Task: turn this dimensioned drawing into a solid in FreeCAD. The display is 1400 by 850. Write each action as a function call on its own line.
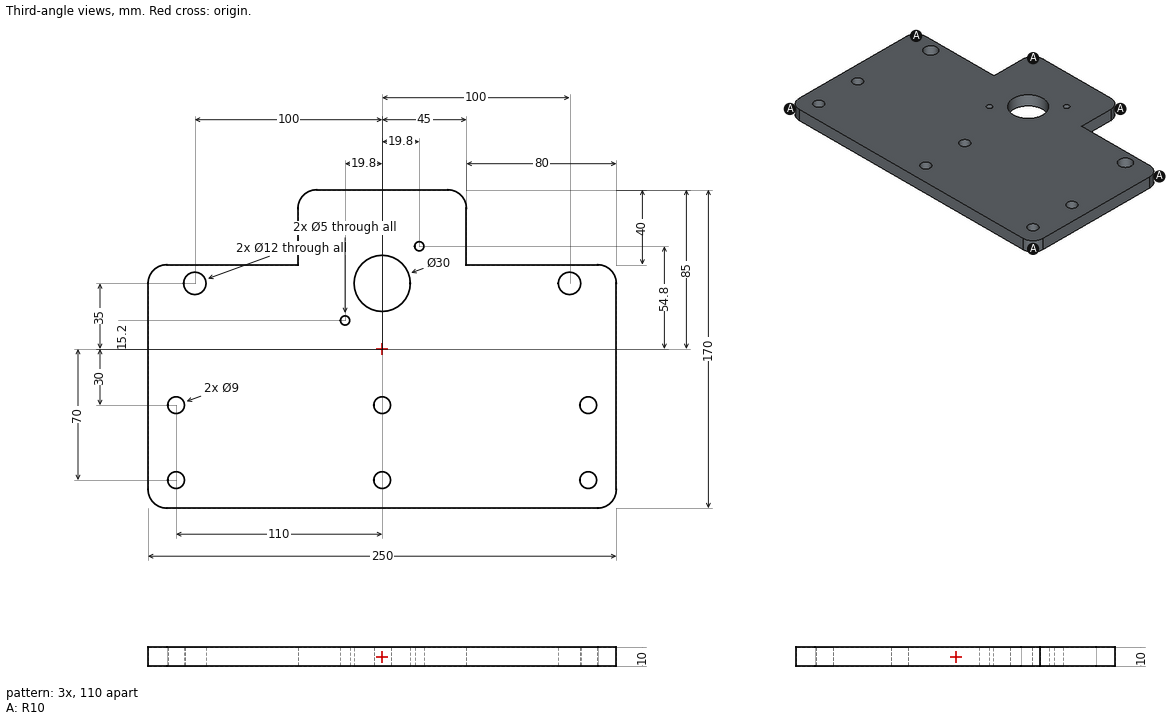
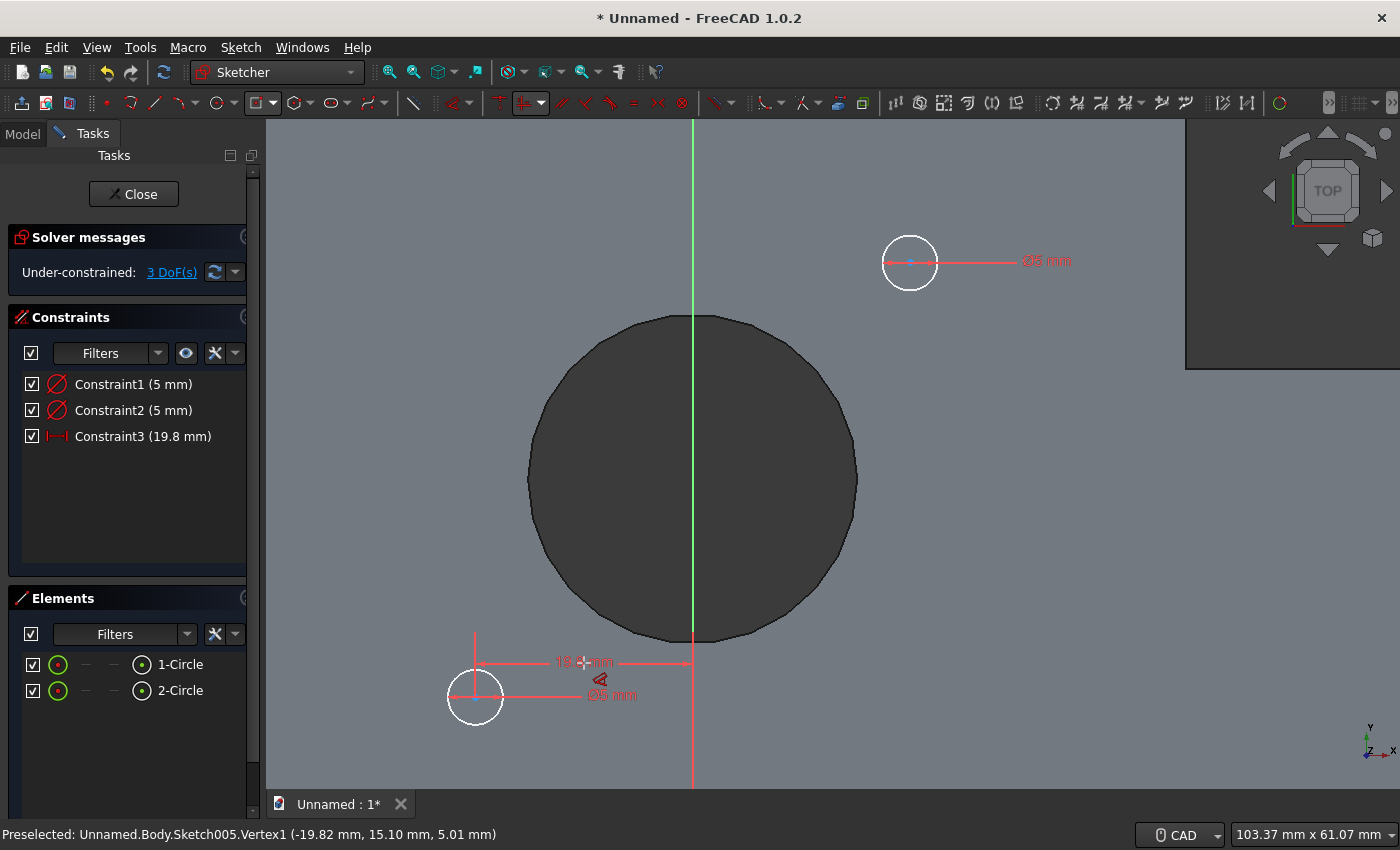
click(475, 697)
click(441, 729)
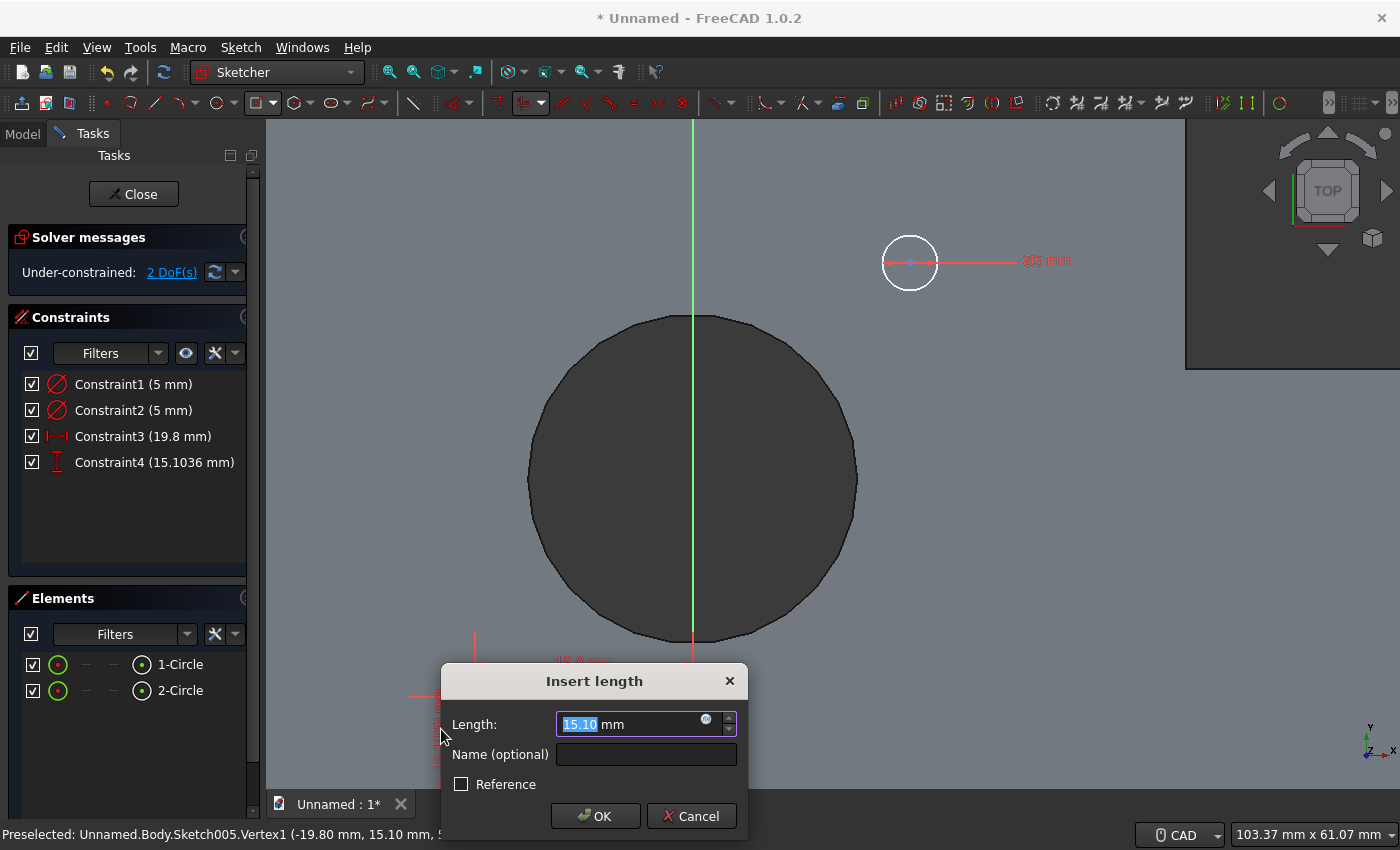
text(15.2)
key(Return)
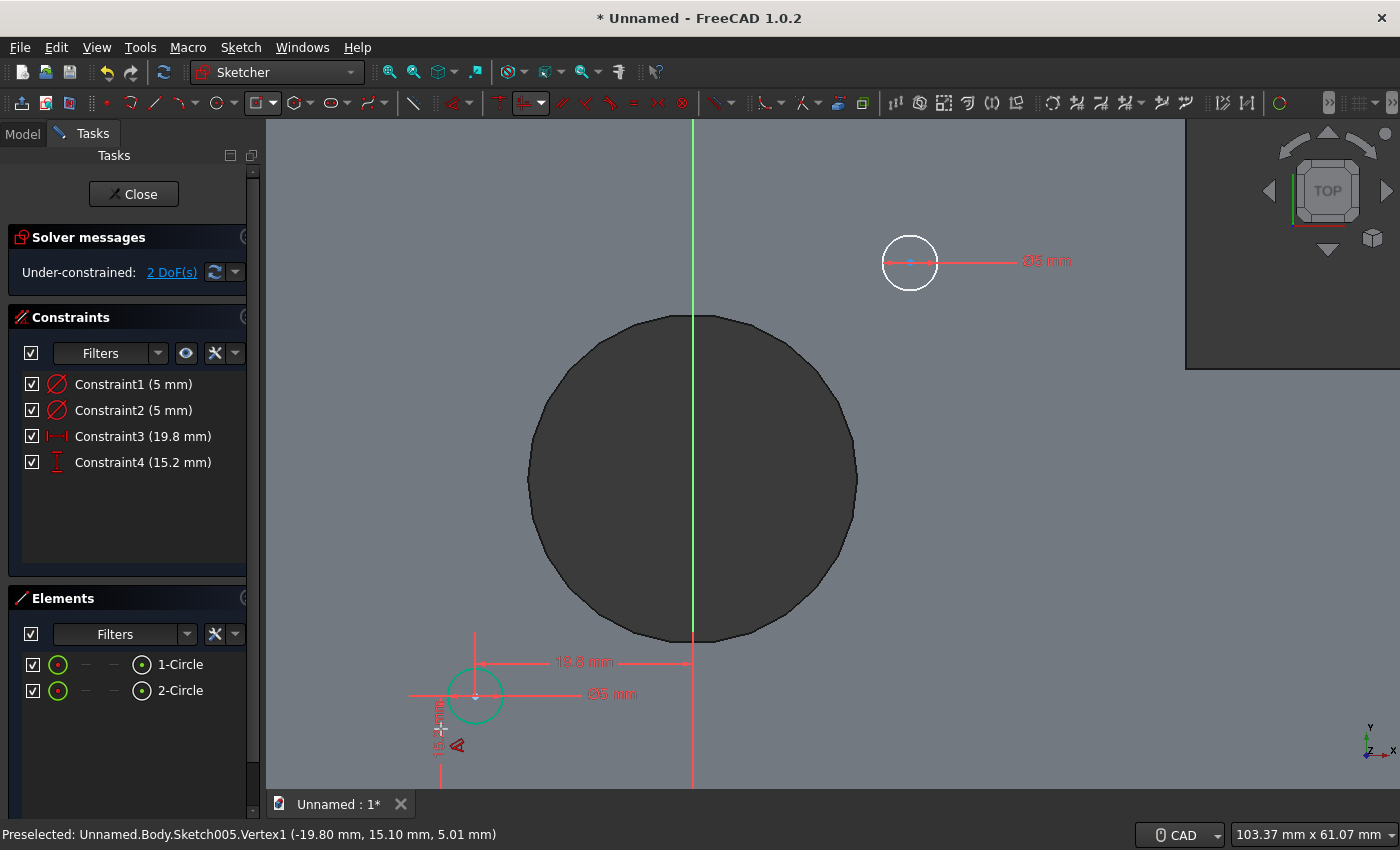
click(910, 263)
click(801, 229)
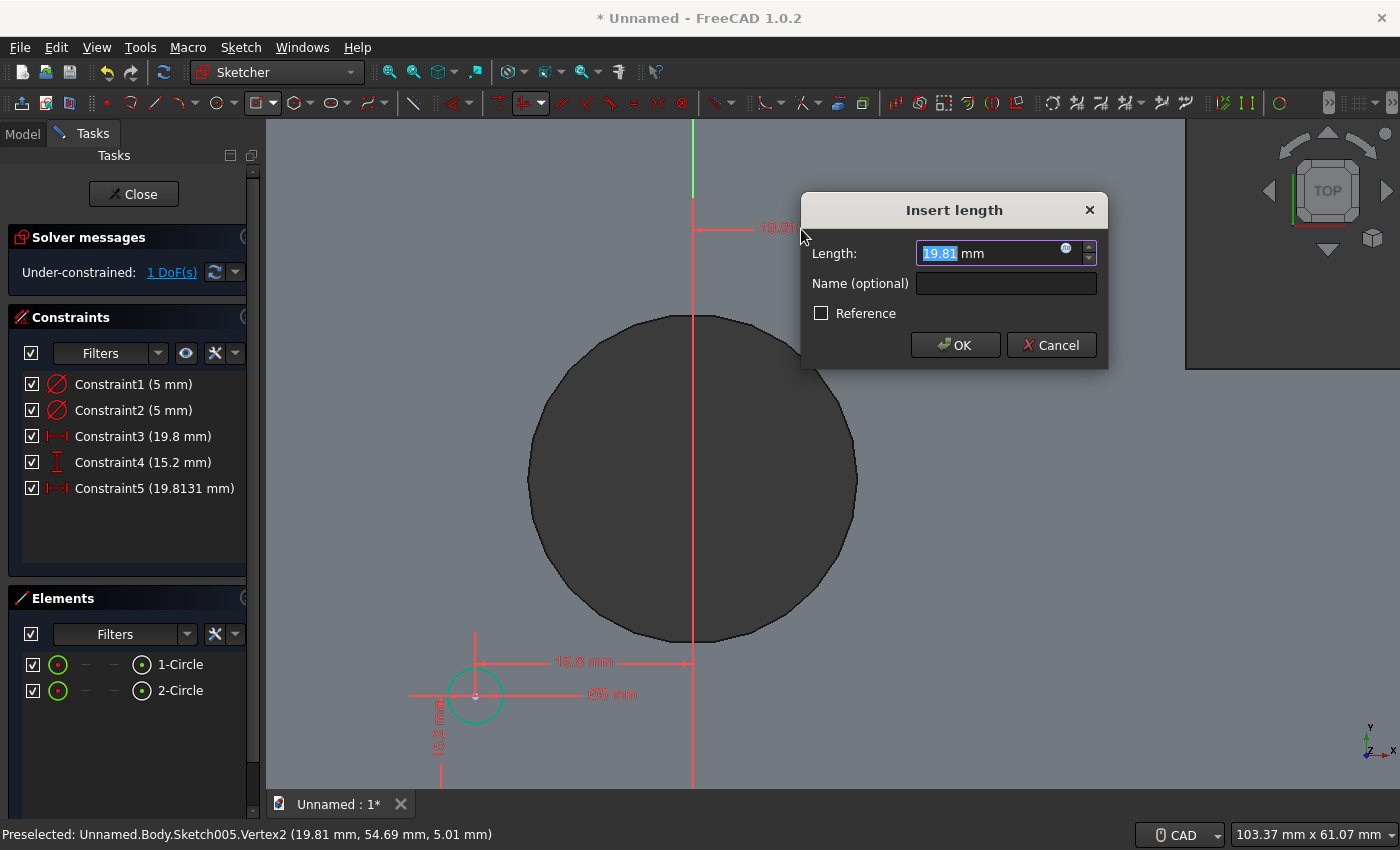
text(19.8)
key(Return)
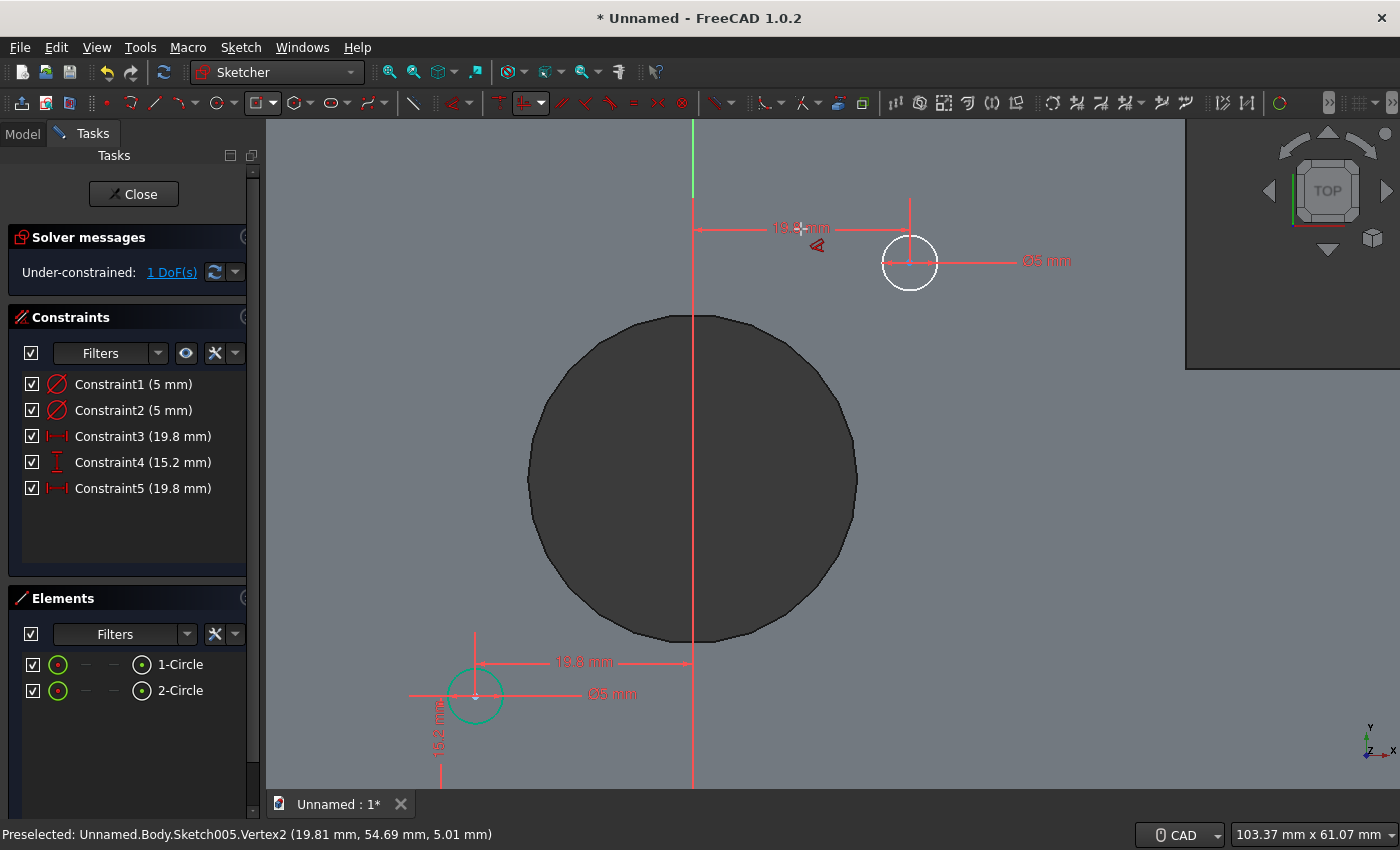
click(910, 263)
click(944, 512)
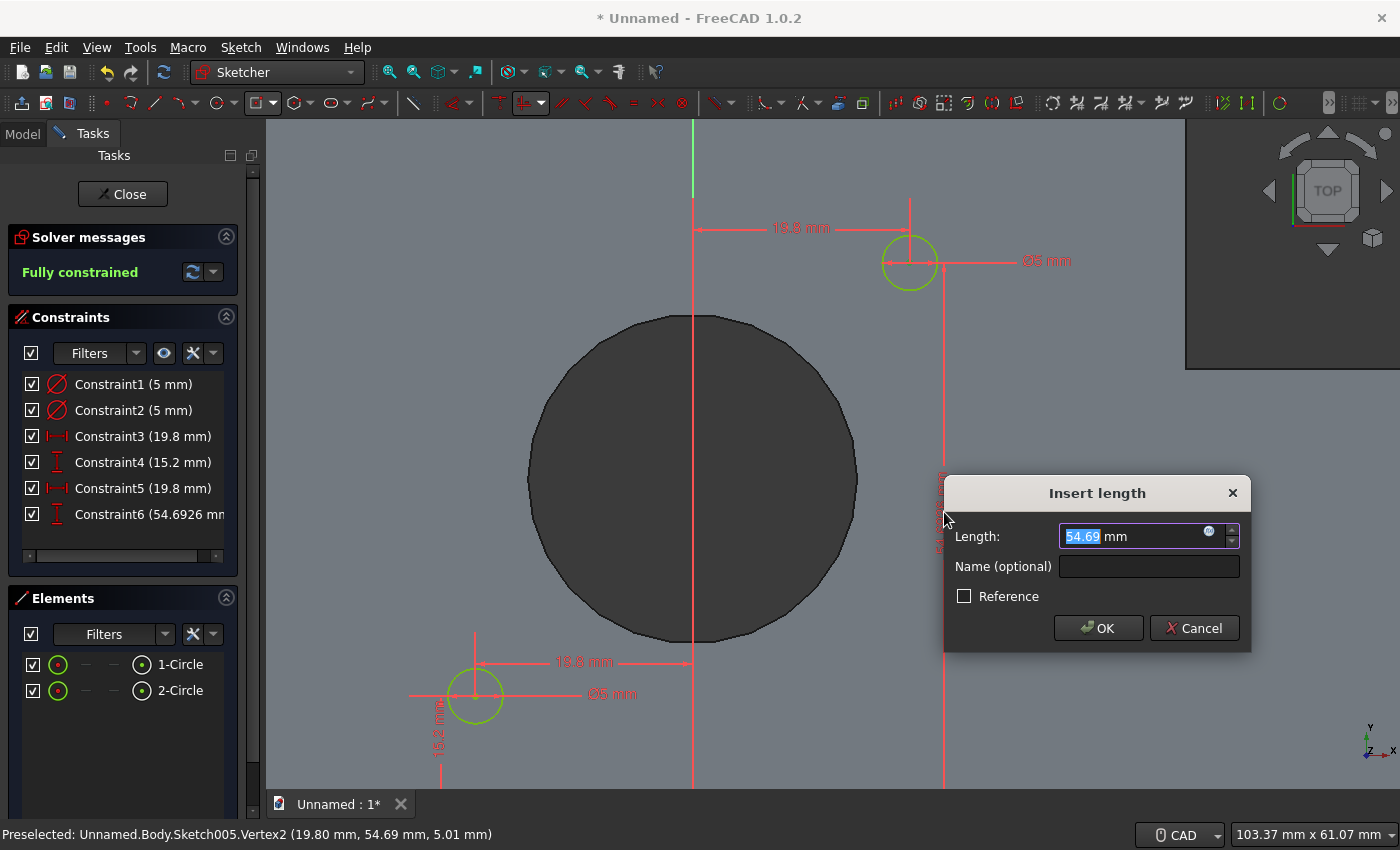
text(54.8)
key(Return)
key(Escape)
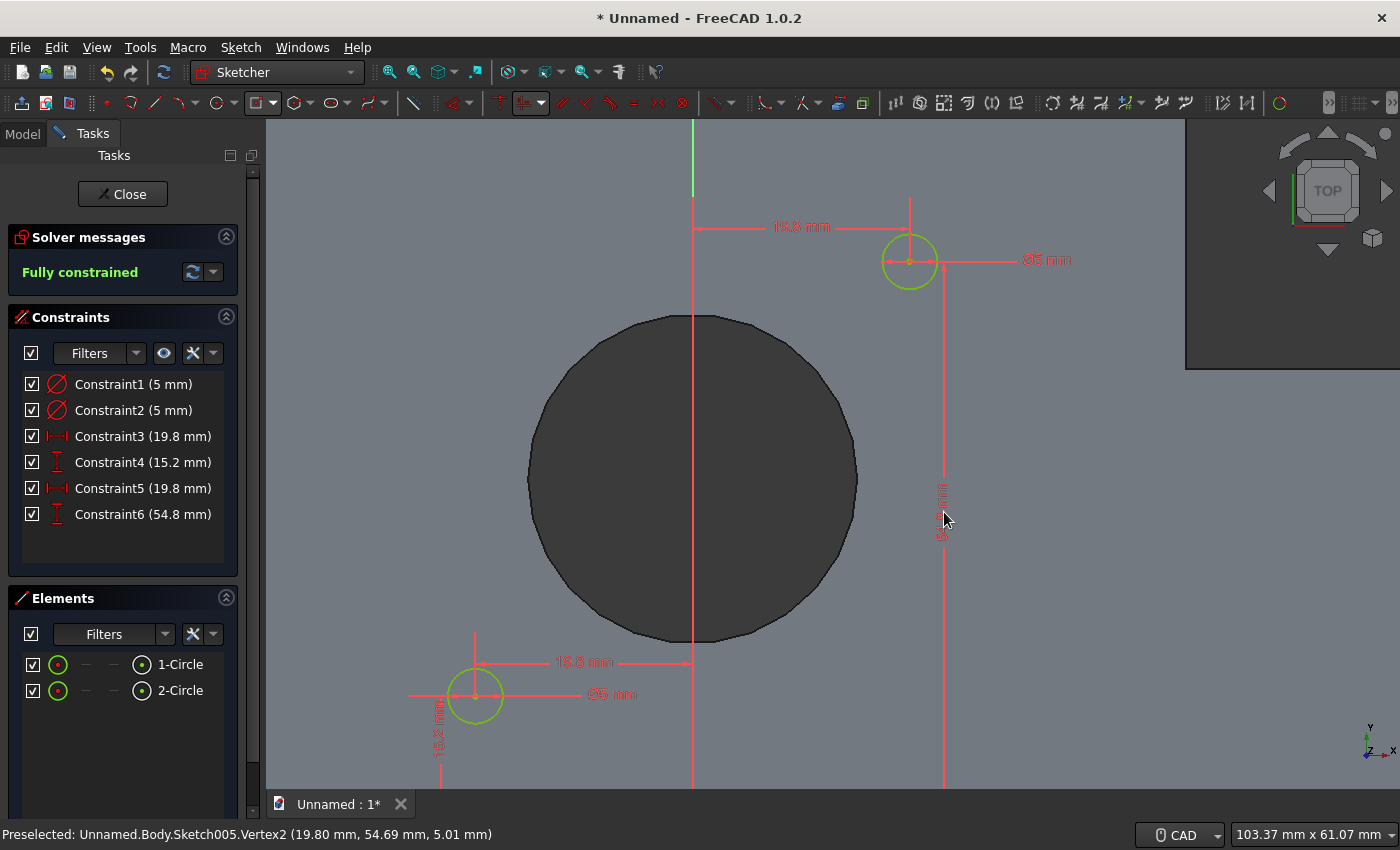
click(123, 194)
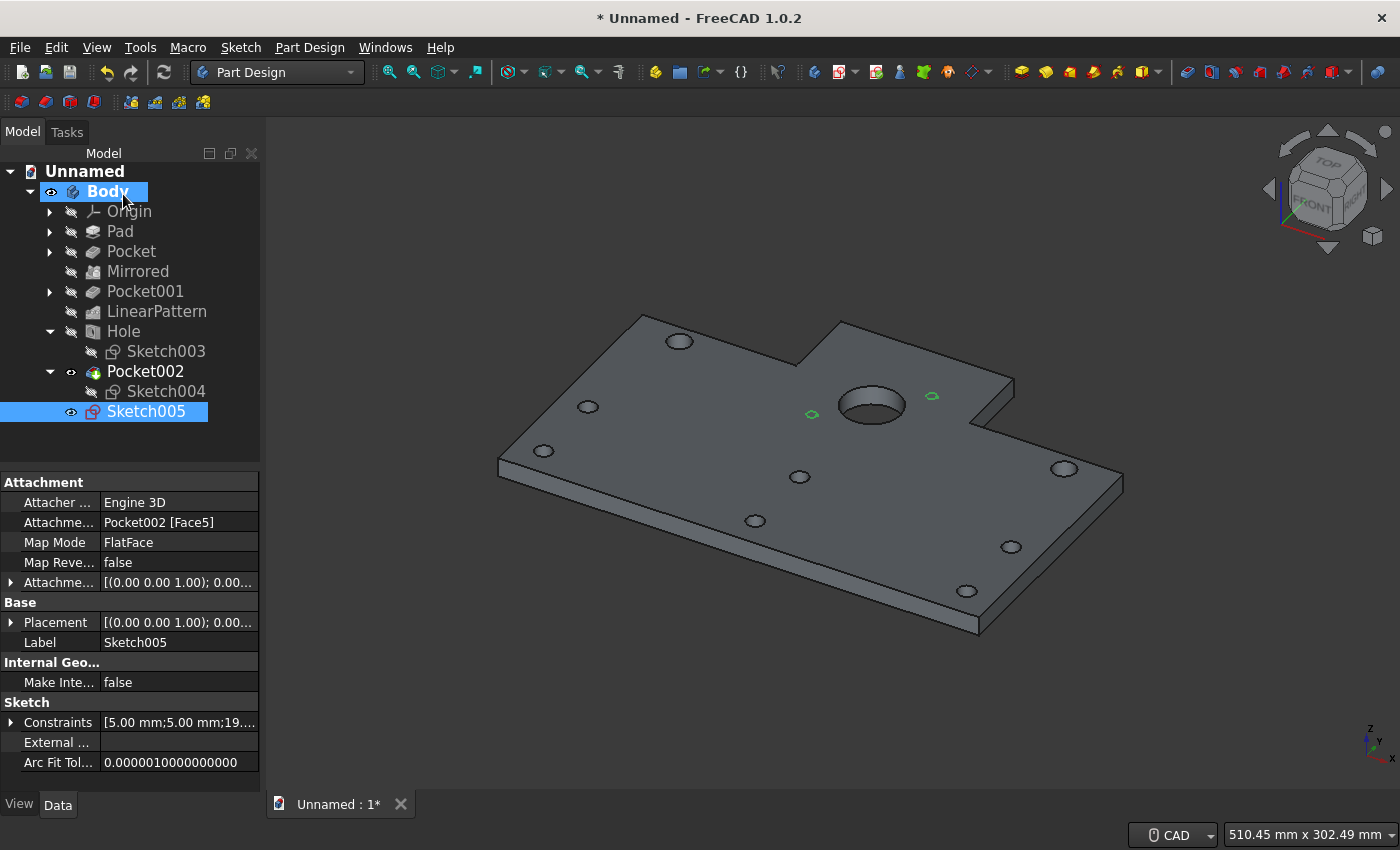
click(1212, 72)